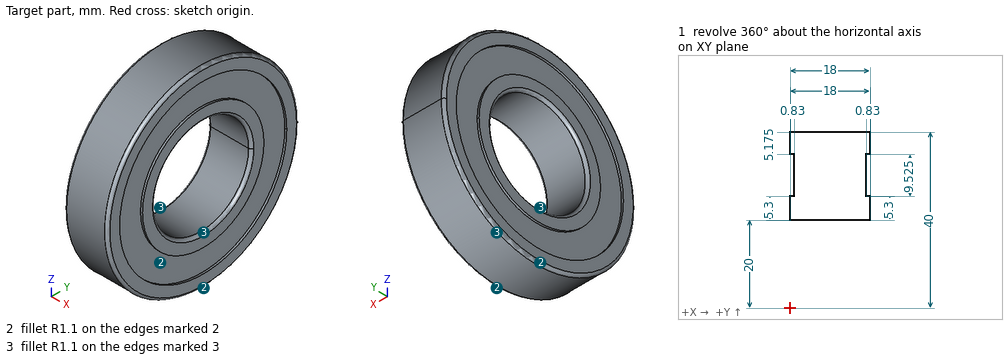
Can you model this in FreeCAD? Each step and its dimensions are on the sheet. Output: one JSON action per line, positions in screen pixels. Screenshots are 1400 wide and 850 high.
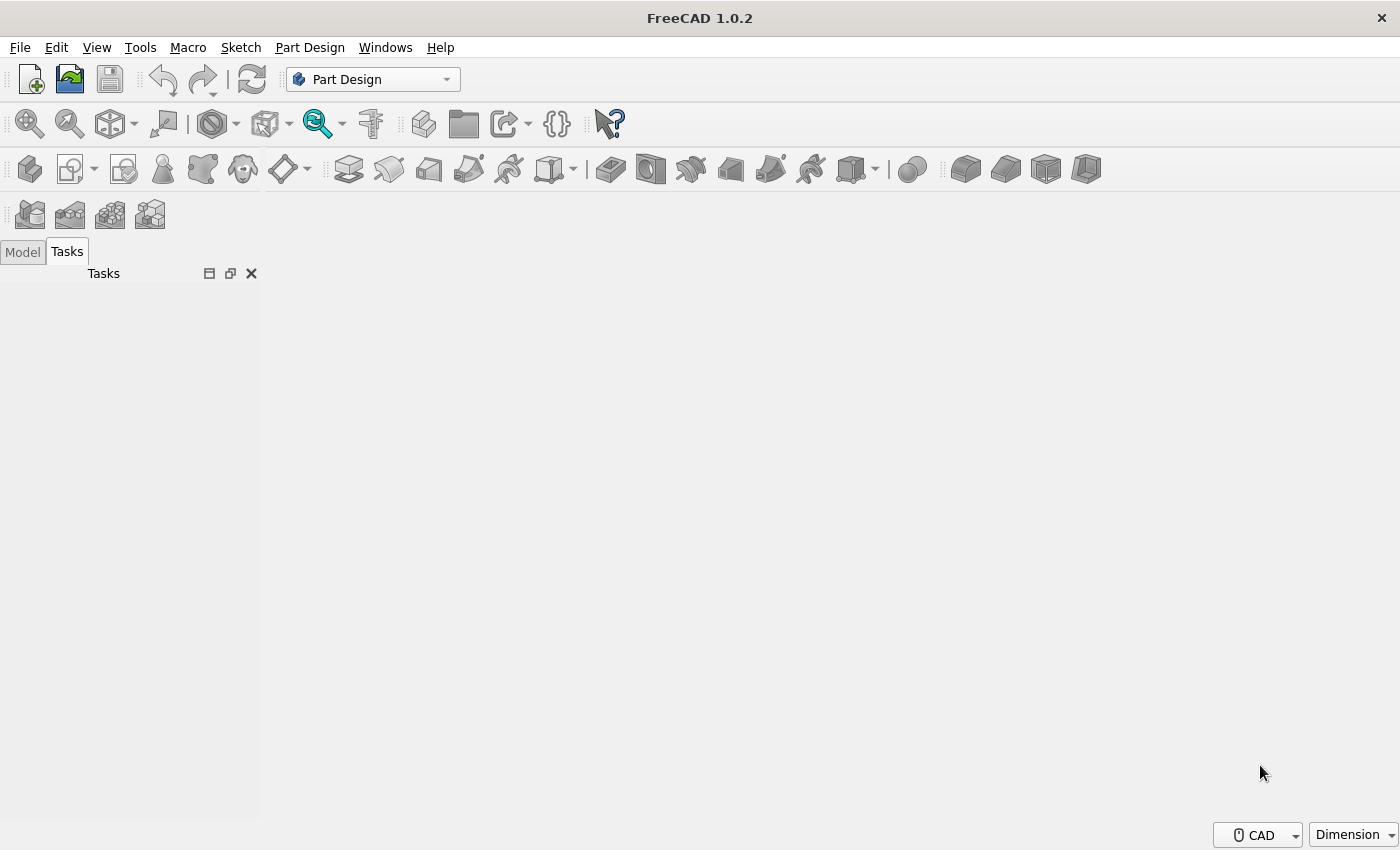
{"action": "left_click", "coordinate": [30, 80]}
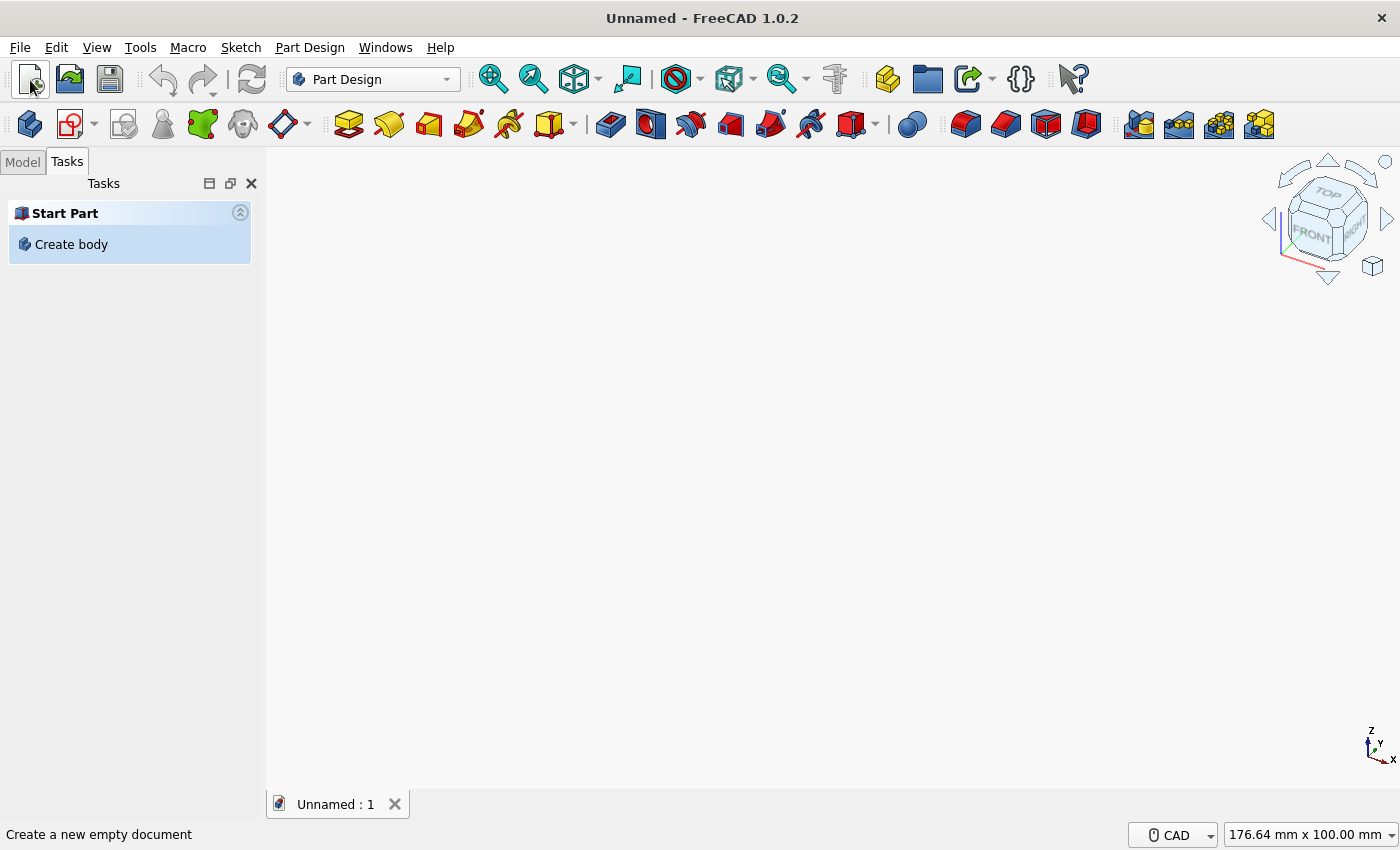
{"action": "left_click", "coordinate": [70, 124]}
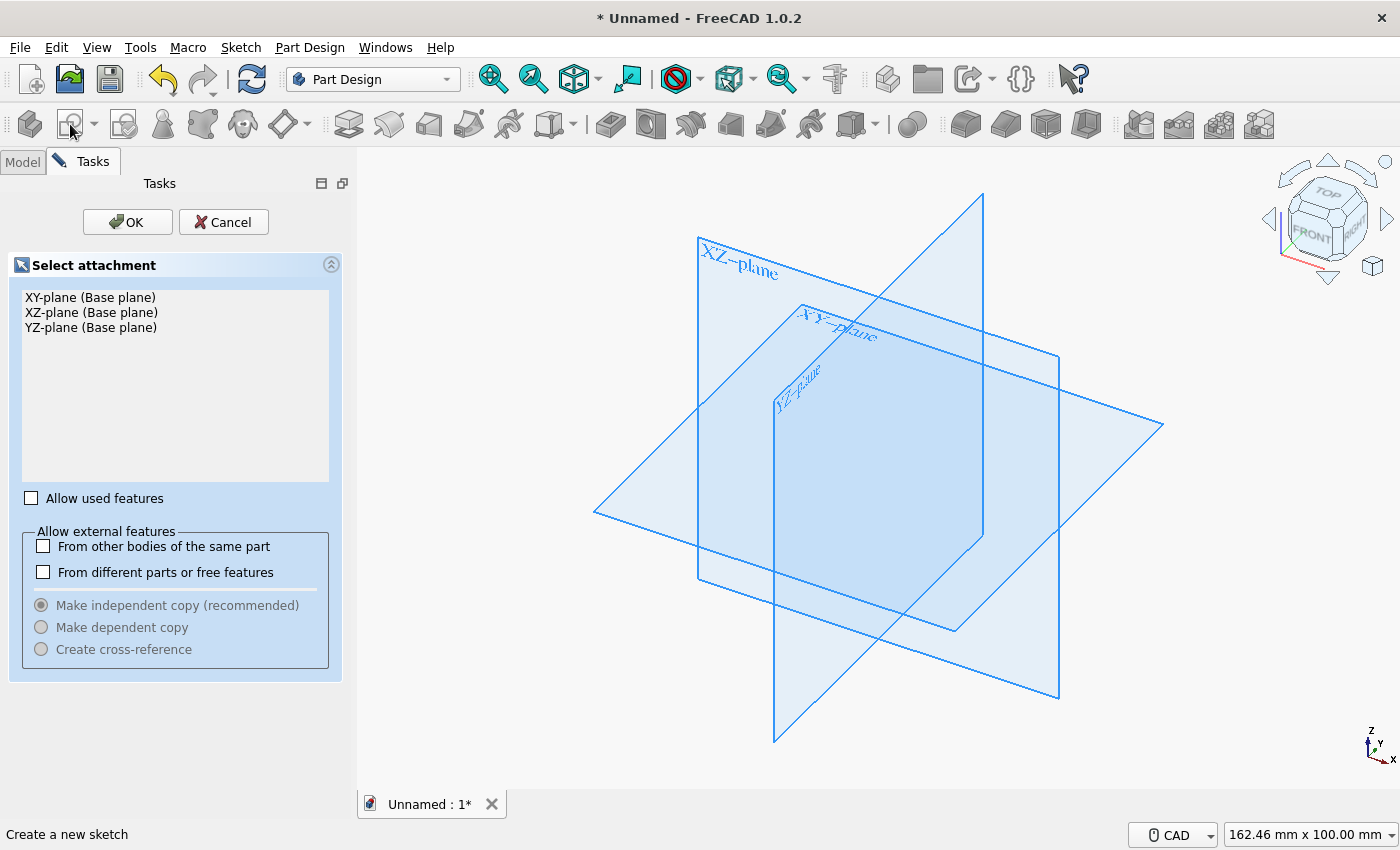
{"action": "left_click", "coordinate": [82, 298]}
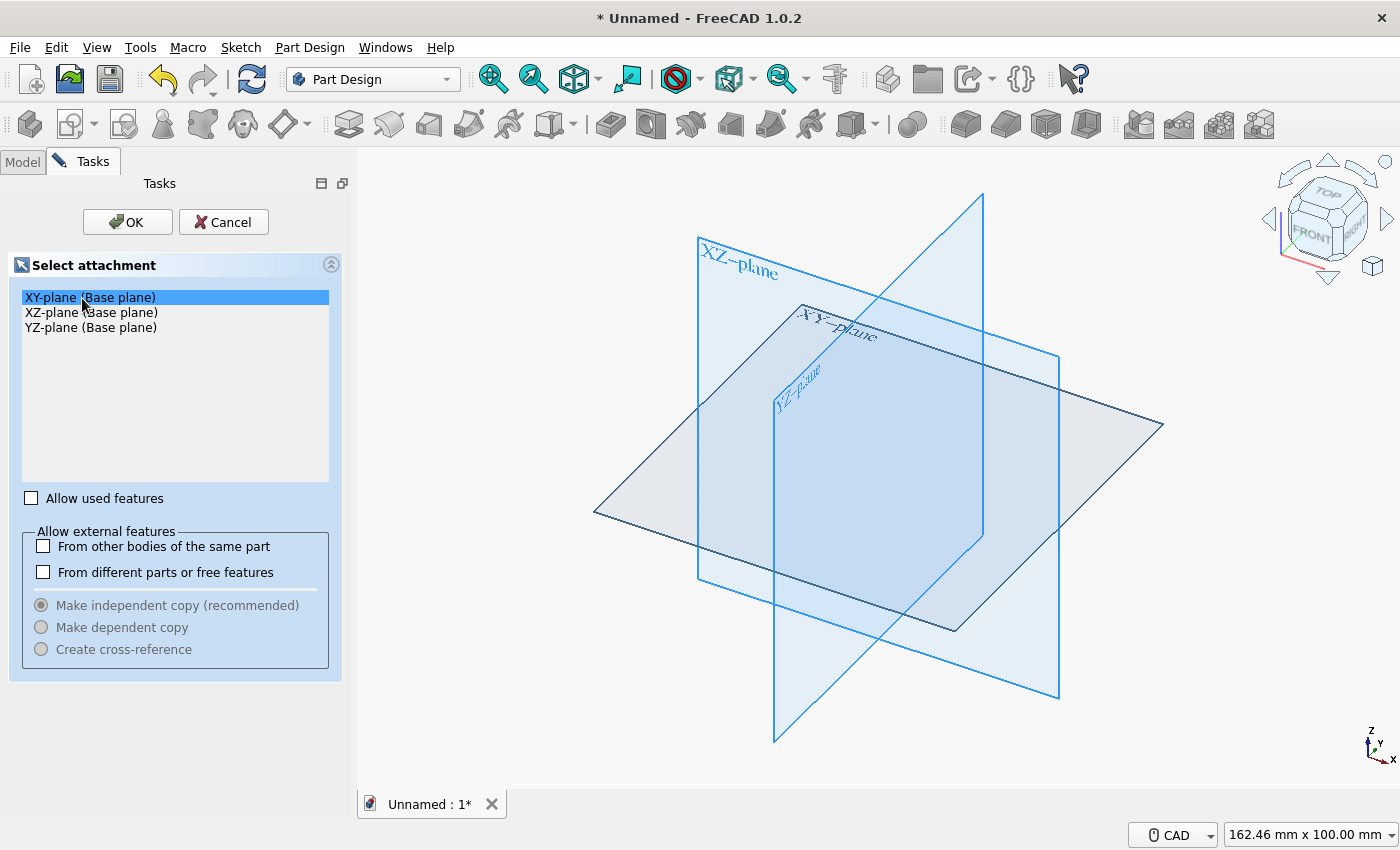
{"action": "left_click", "coordinate": [128, 222]}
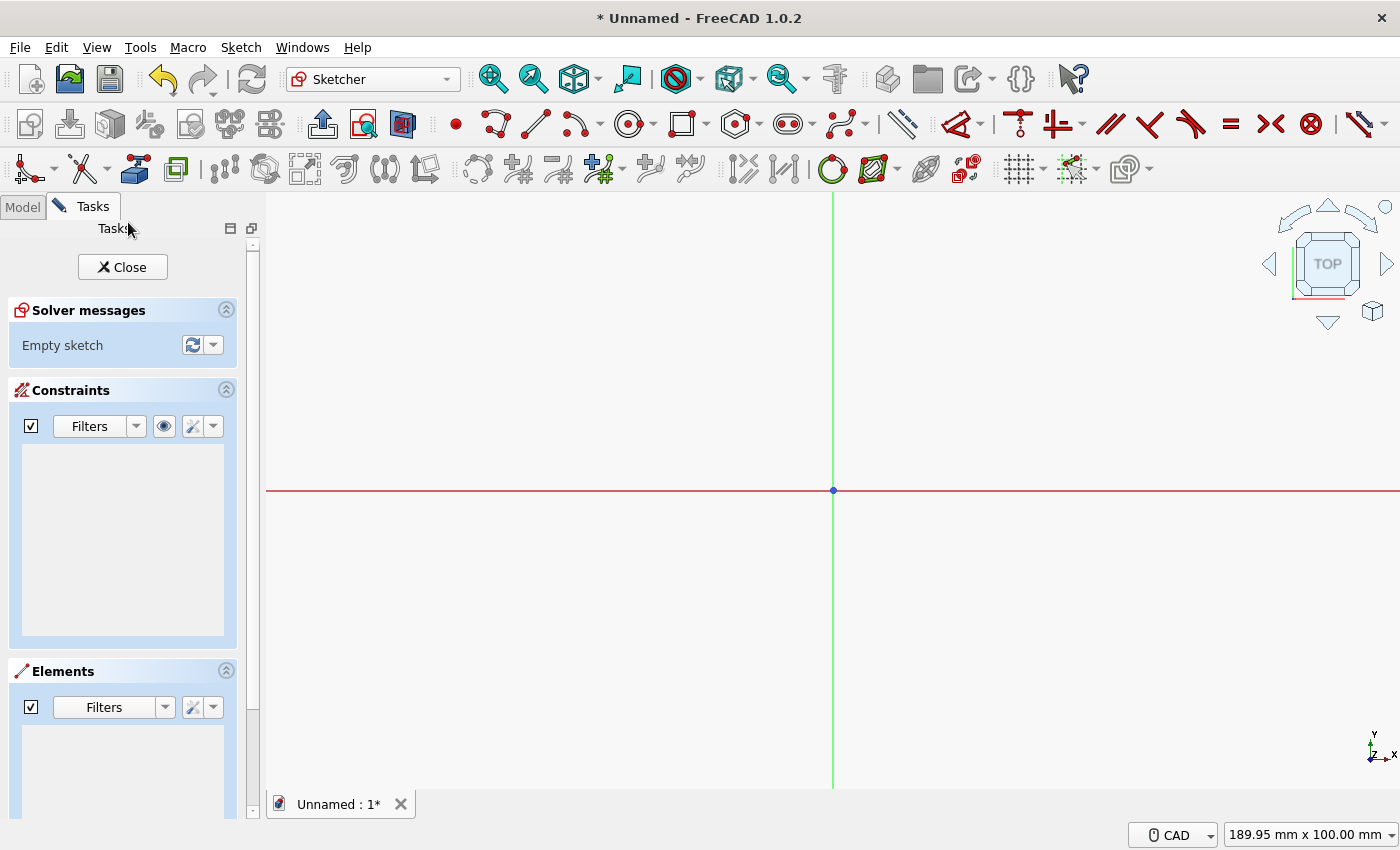
{"action": "scroll", "coordinate": [1135, 220], "scroll_direction": "up", "scroll_amount": 2}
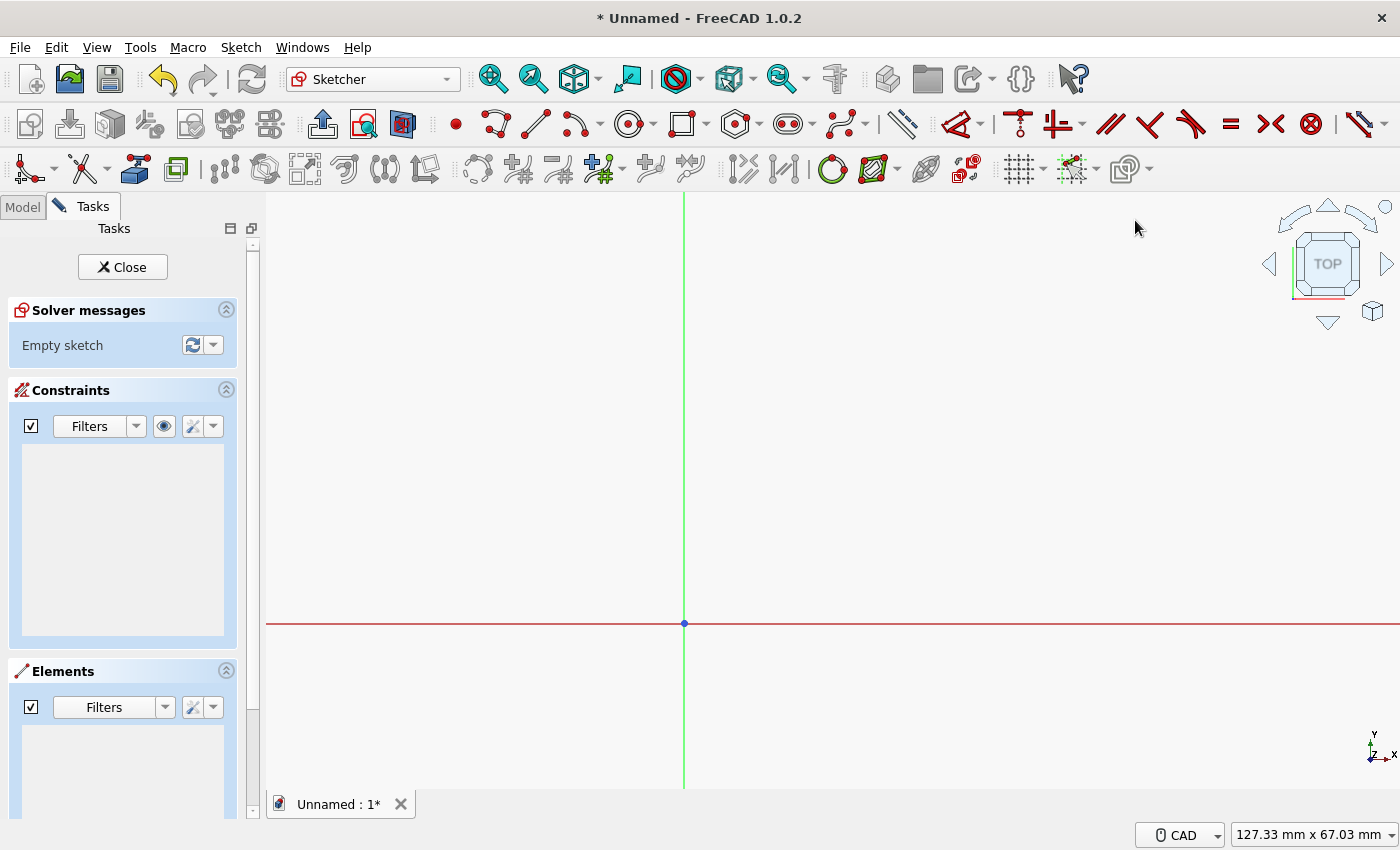
{"action": "left_click", "coordinate": [496, 124]}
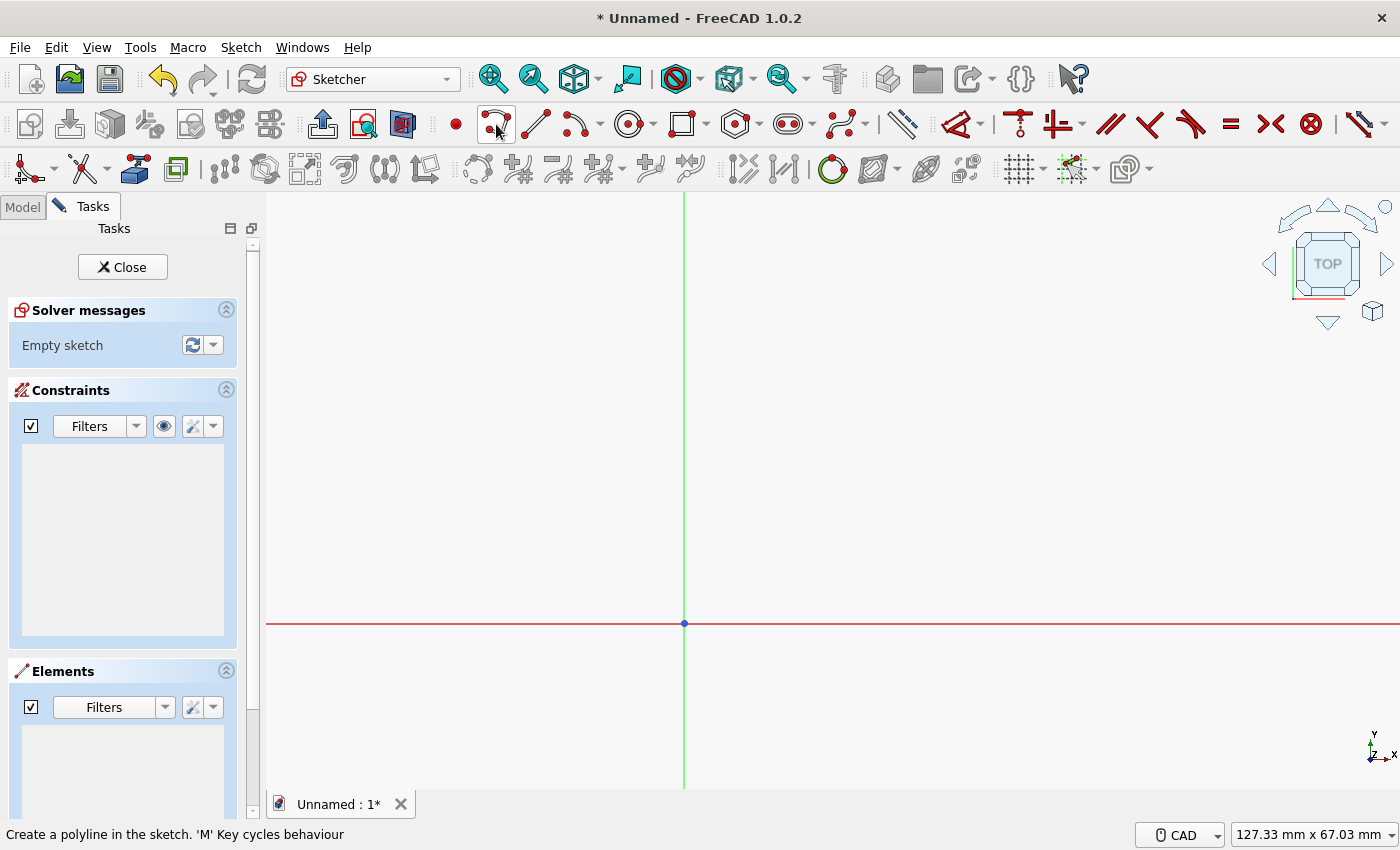
{"action": "left_click", "coordinate": [684, 445]}
{"action": "left_click", "coordinate": [844, 445]}
{"action": "left_click", "coordinate": [844, 398]}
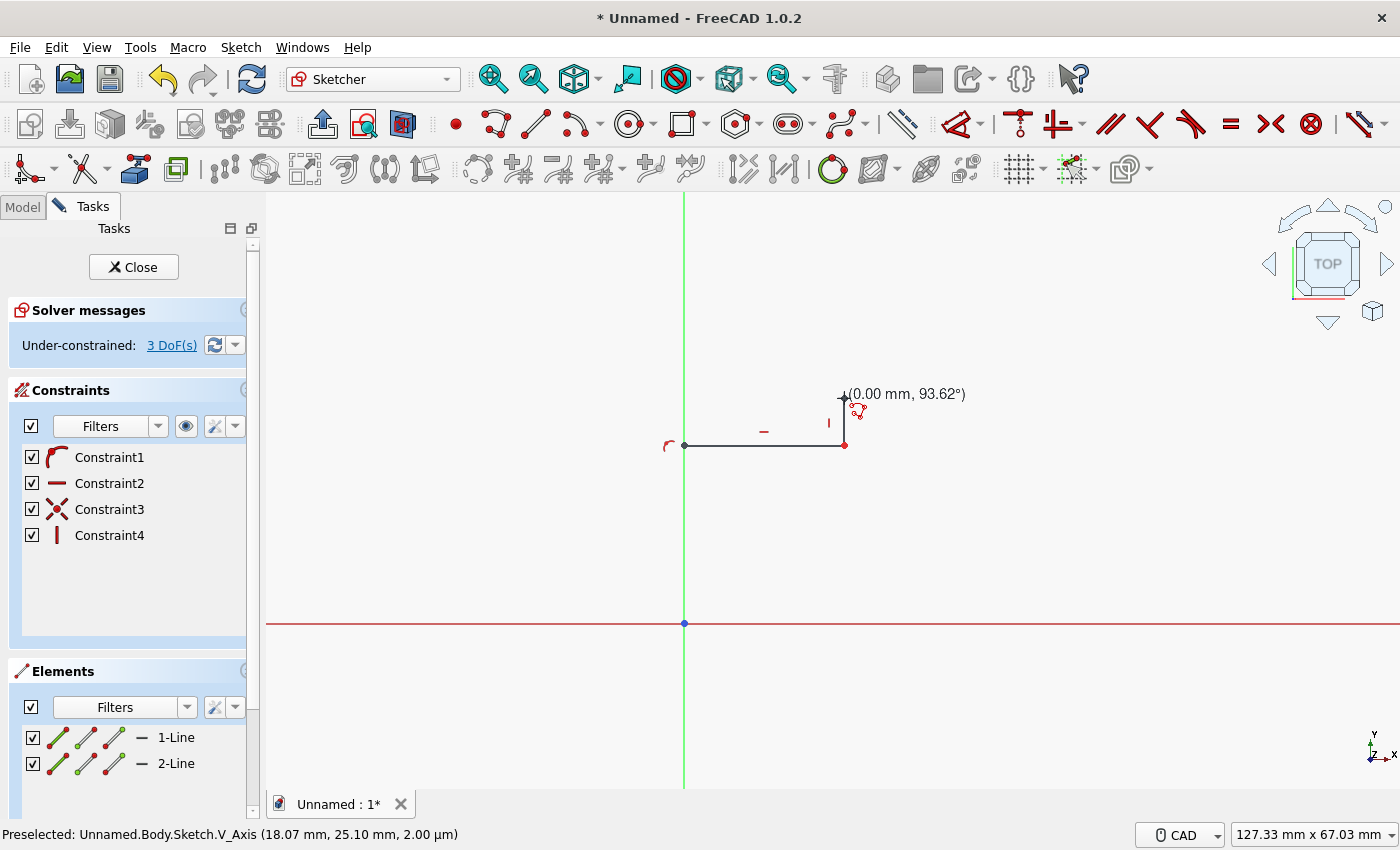
{"action": "scroll", "coordinate": [837, 398], "scroll_direction": "up", "scroll_amount": 4}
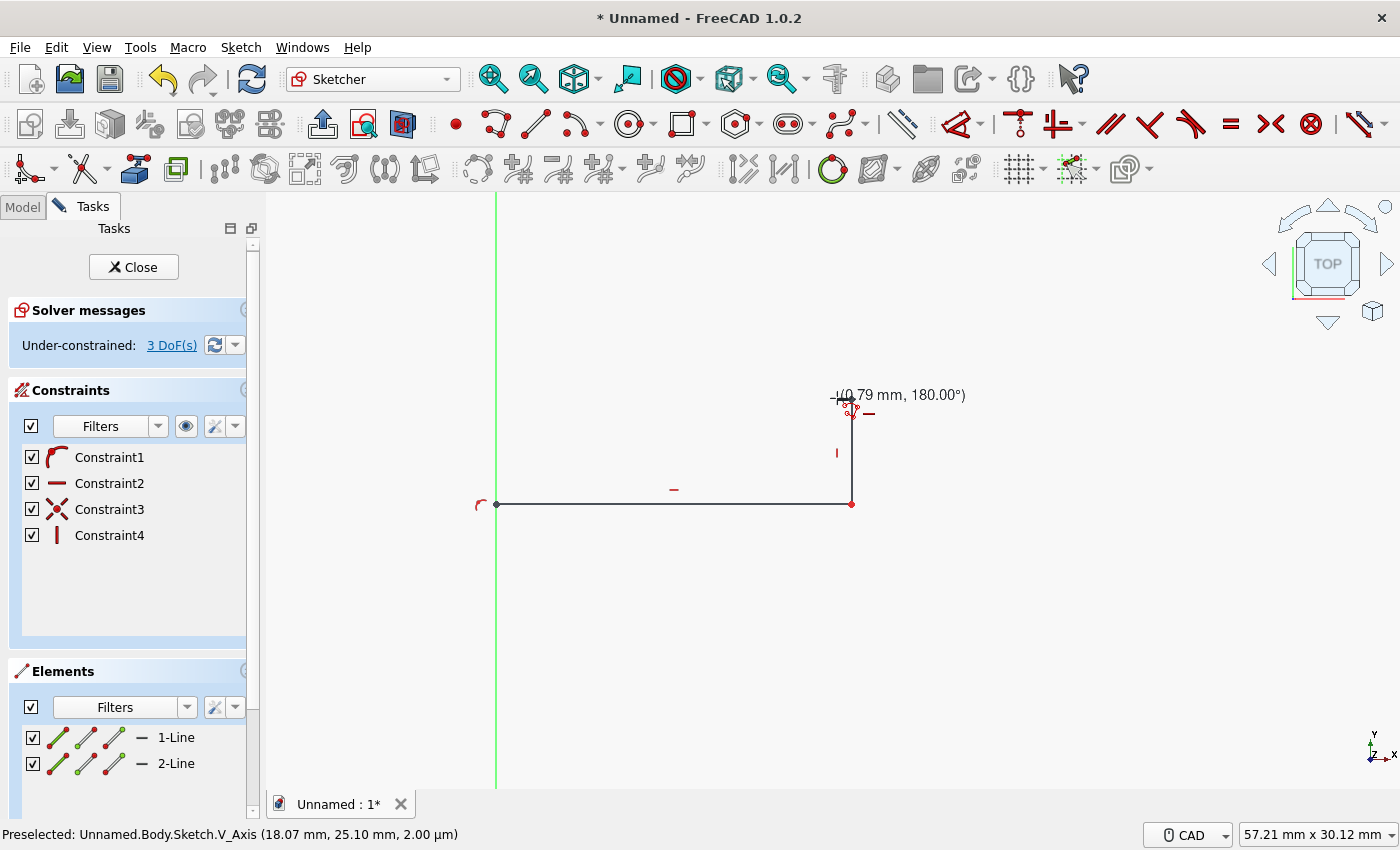
{"action": "left_click", "coordinate": [836, 398]}